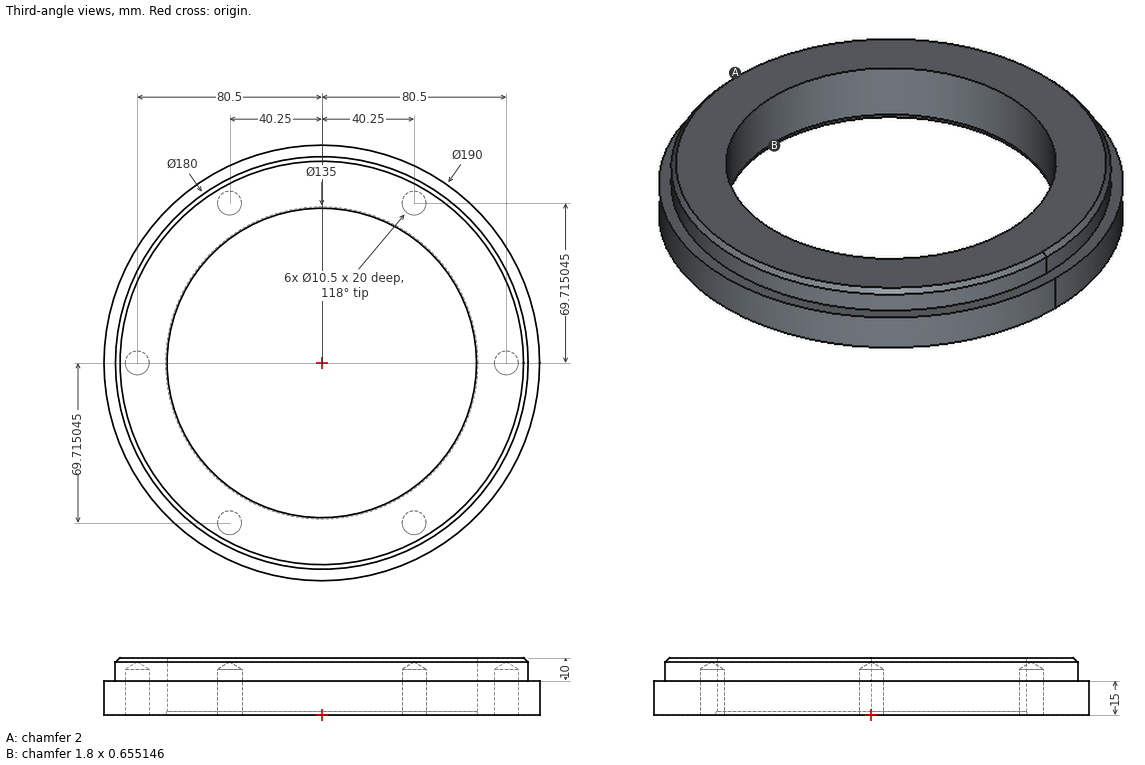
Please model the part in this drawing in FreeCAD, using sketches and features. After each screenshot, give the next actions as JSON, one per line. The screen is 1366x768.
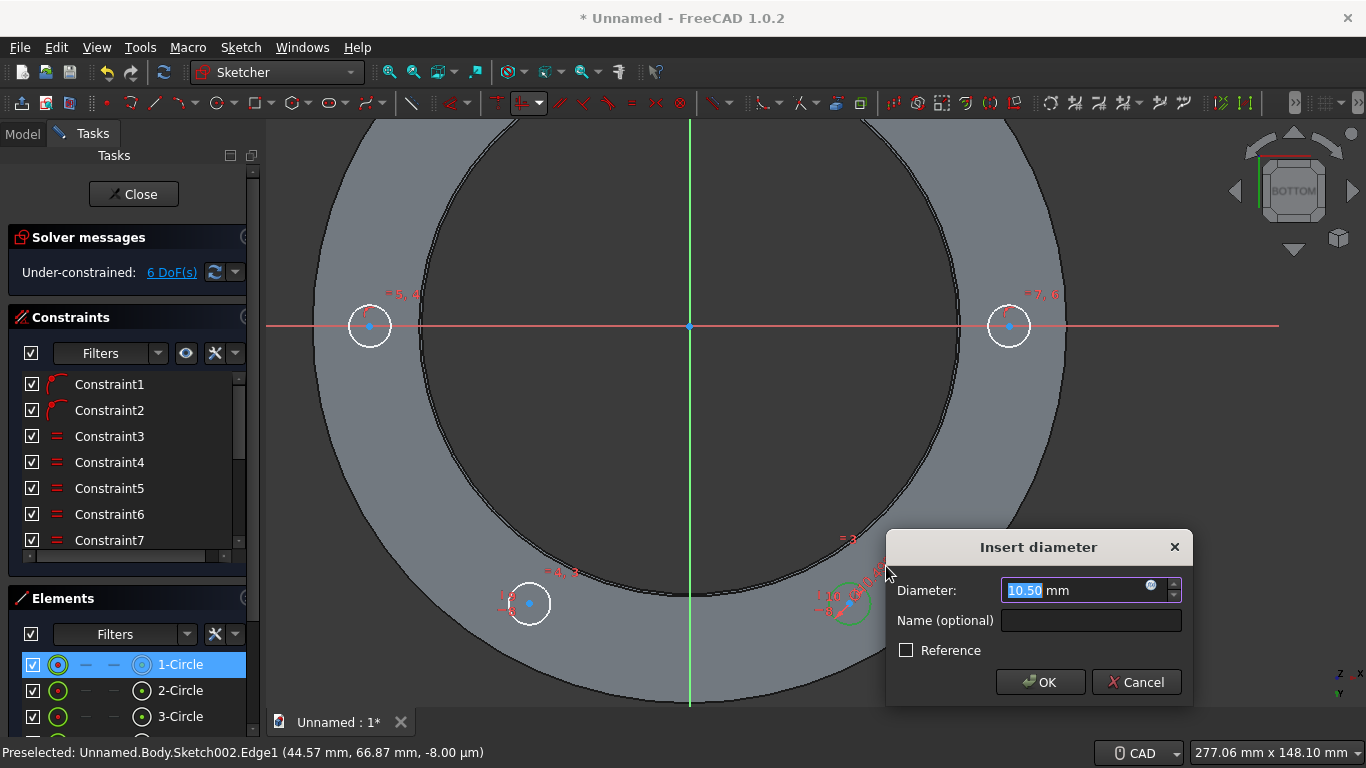
{"action": "type", "text": "10.5"}
{"action": "key", "text": "Return"}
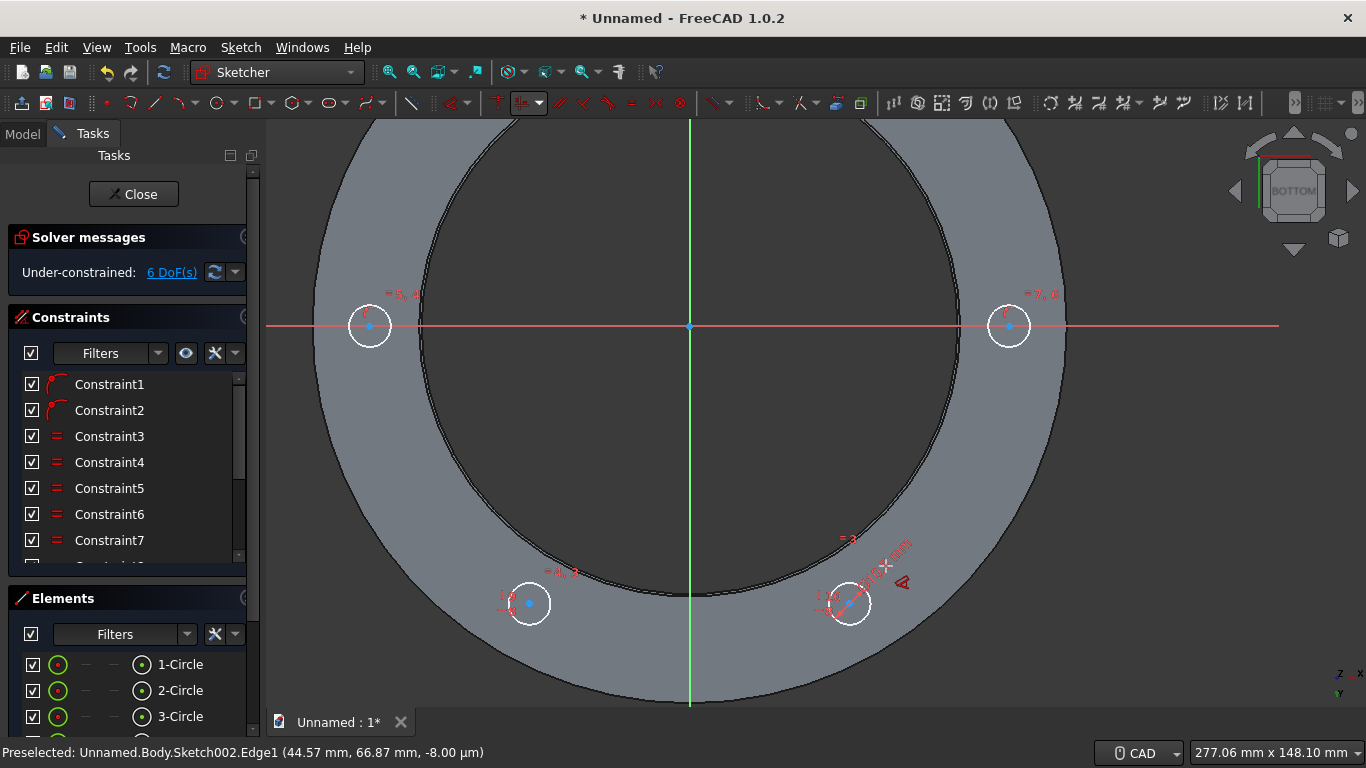
{"action": "left_click", "coordinate": [370, 326]}
{"action": "left_click", "coordinate": [530, 360]}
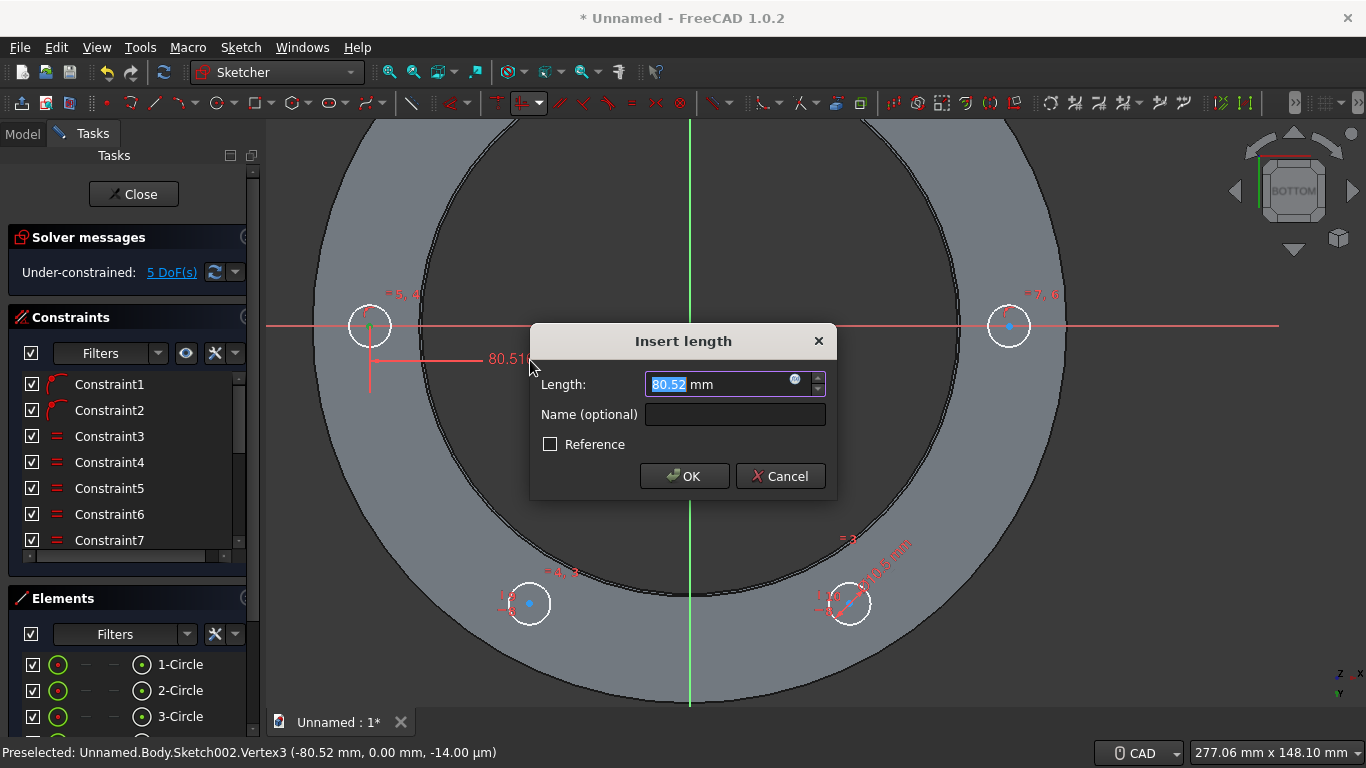
{"action": "type", "text": "80.5"}
{"action": "key", "text": "Return"}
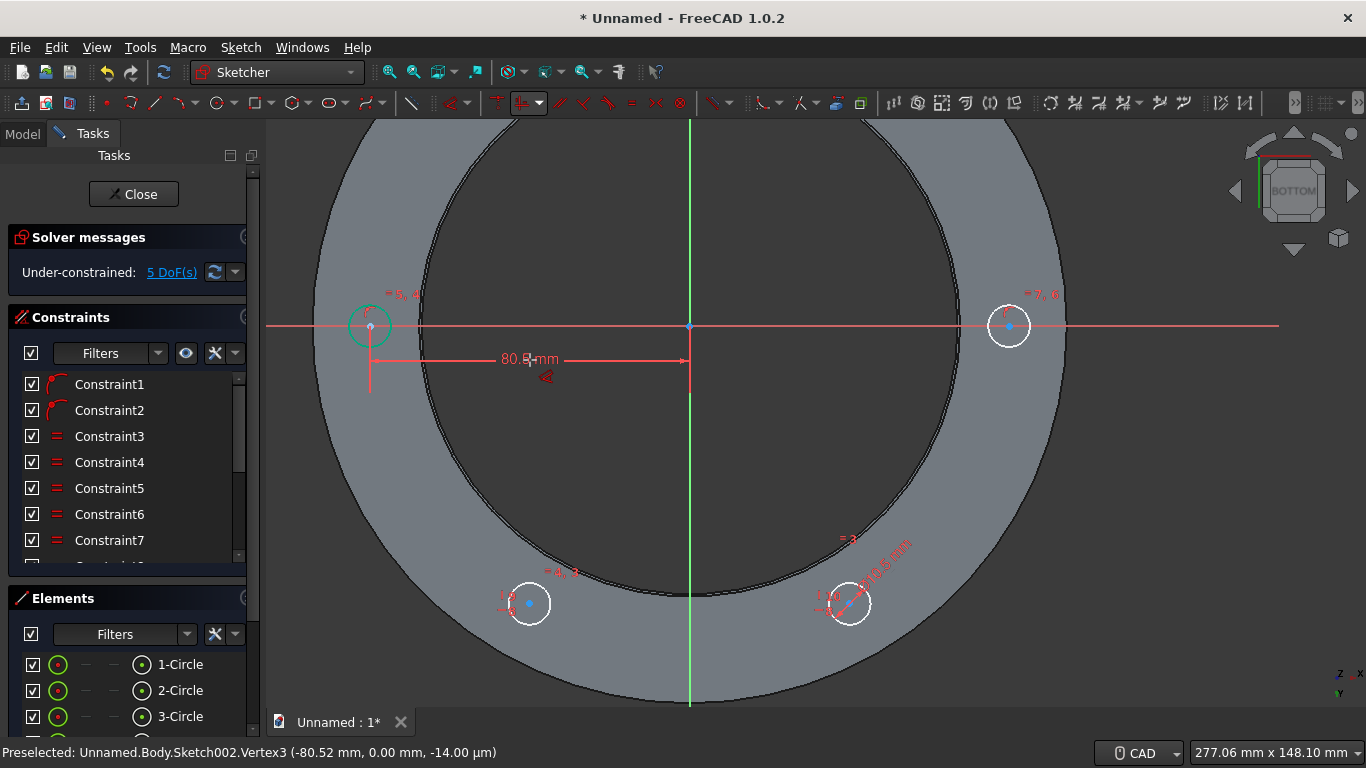
{"action": "left_click", "coordinate": [1009, 326]}
{"action": "left_click", "coordinate": [849, 360]}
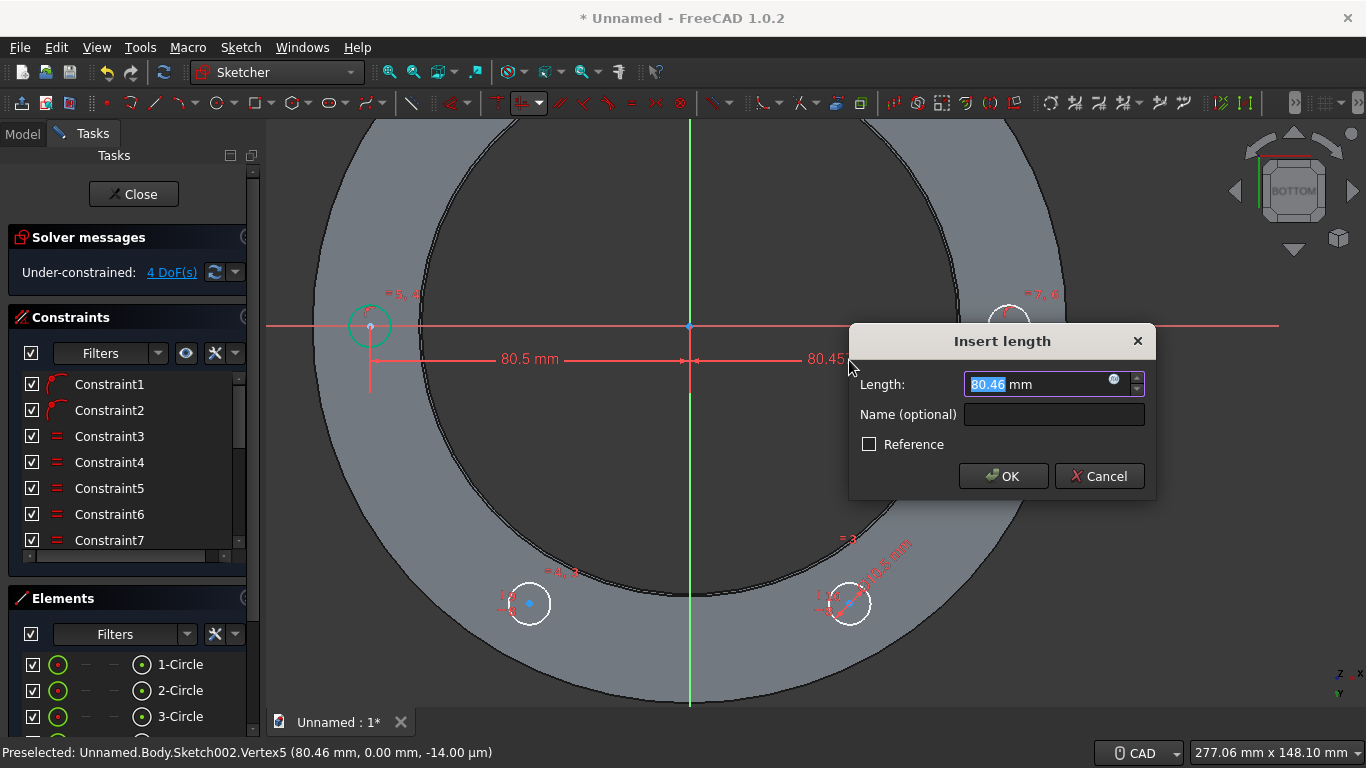
{"action": "type", "text": "80.5"}
{"action": "key", "text": "Return"}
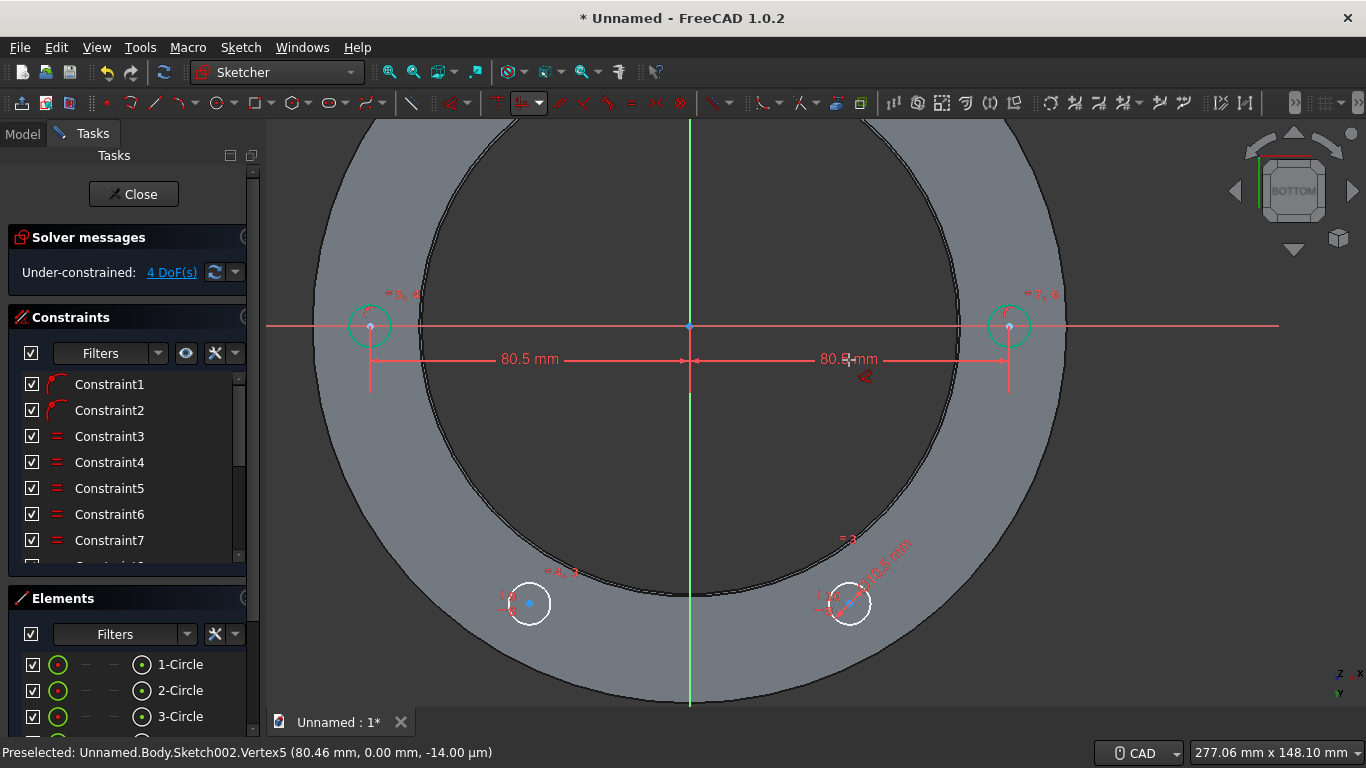
{"action": "left_click", "coordinate": [850, 604]}
{"action": "left_click", "coordinate": [770, 638]}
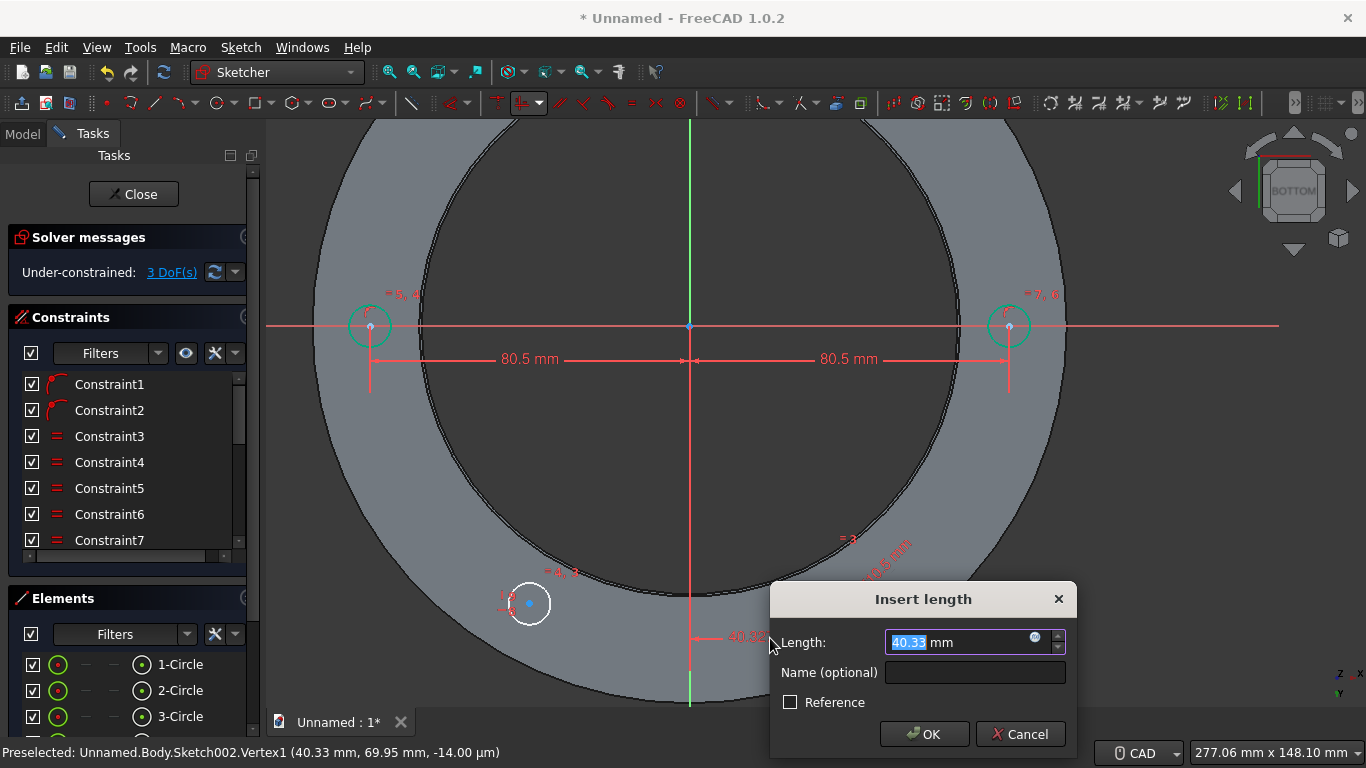
{"action": "type", "text": "40.25"}
{"action": "key", "text": "Return"}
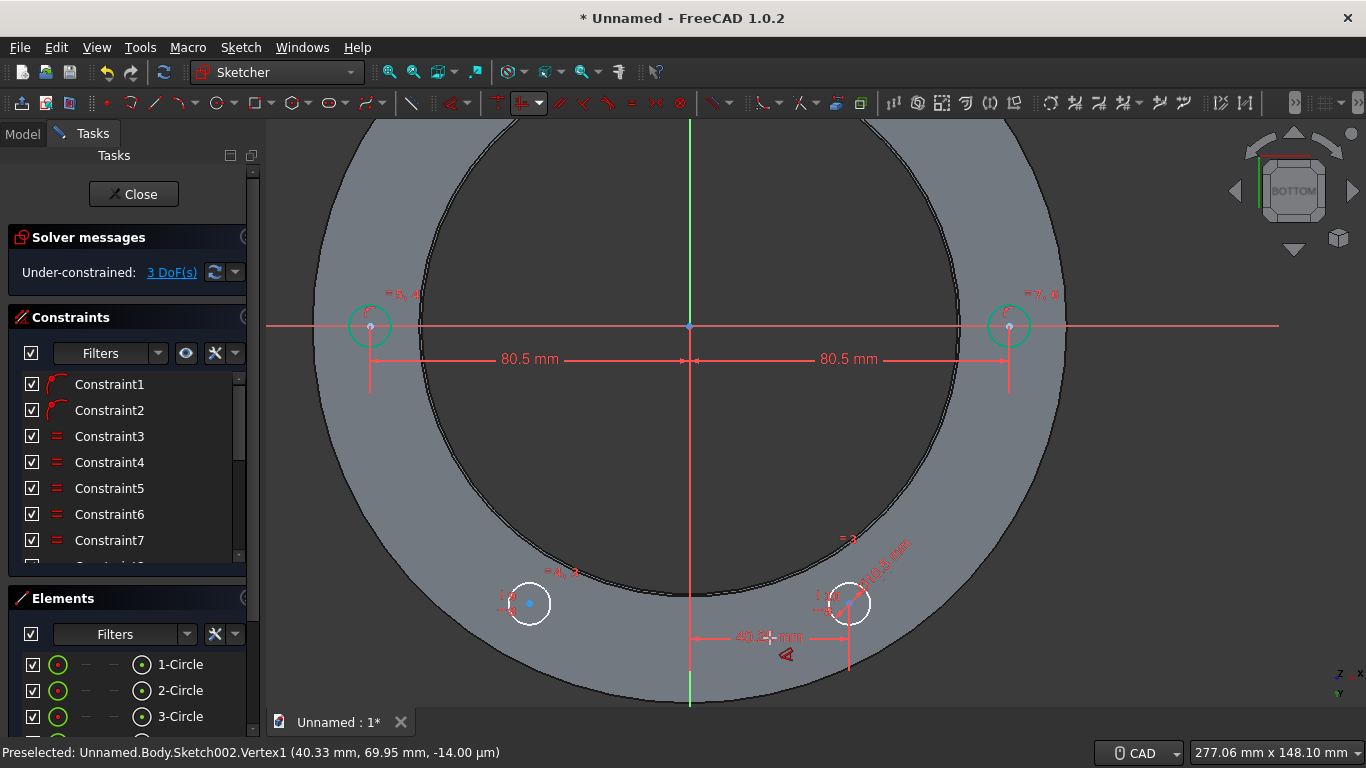
{"action": "left_click", "coordinate": [530, 604]}
{"action": "left_click", "coordinate": [610, 638]}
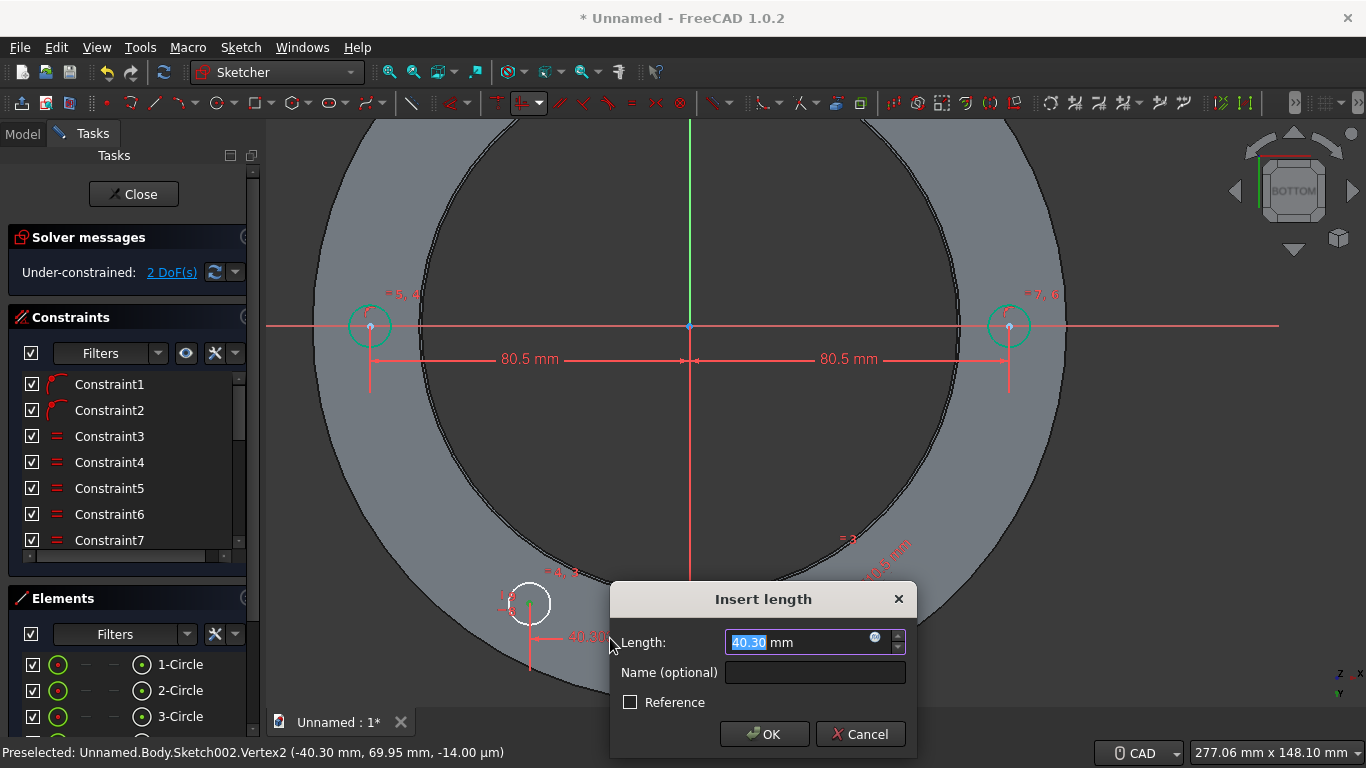
{"action": "type", "text": "40.25"}
{"action": "key", "text": "Return"}